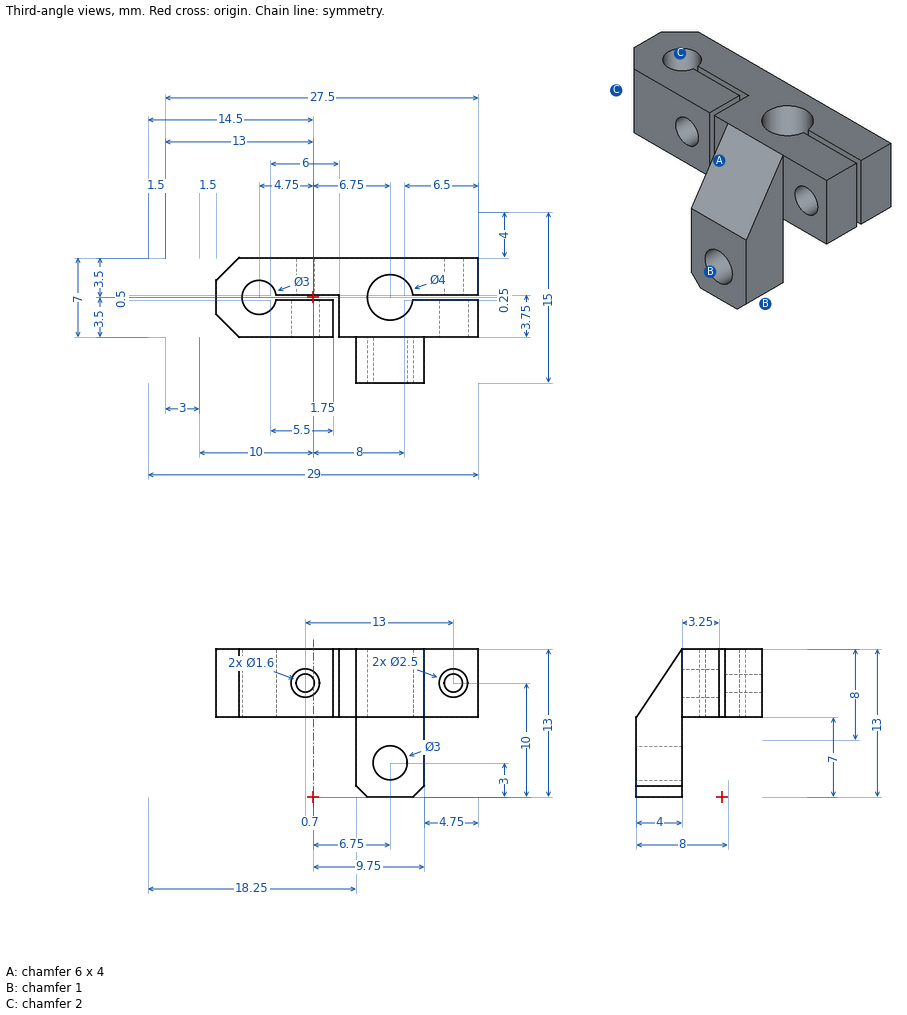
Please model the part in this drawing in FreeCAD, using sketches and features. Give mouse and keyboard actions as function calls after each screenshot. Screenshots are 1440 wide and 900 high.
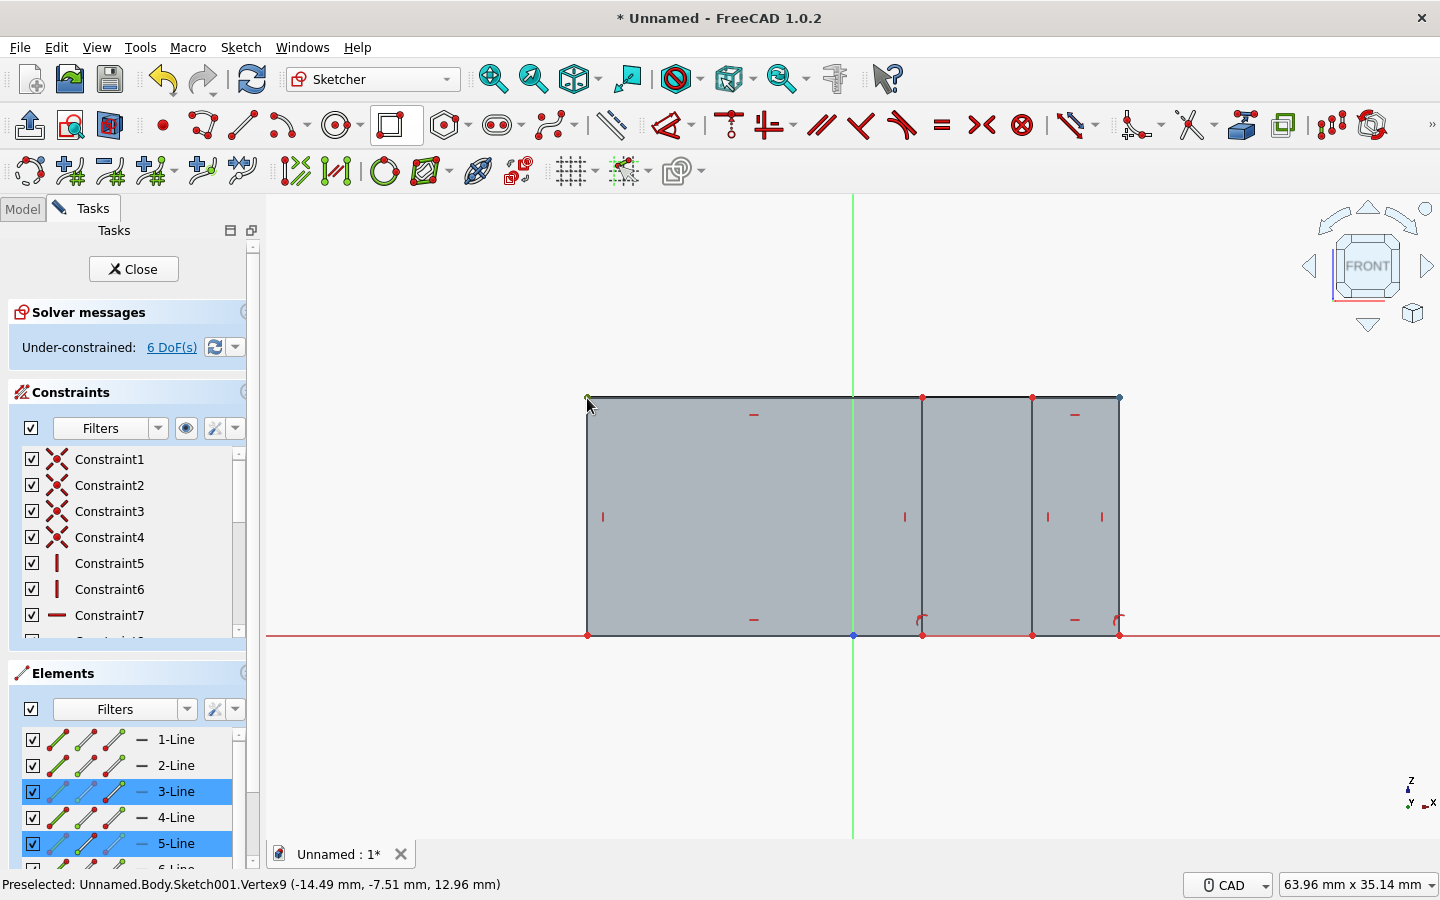
click(853, 769)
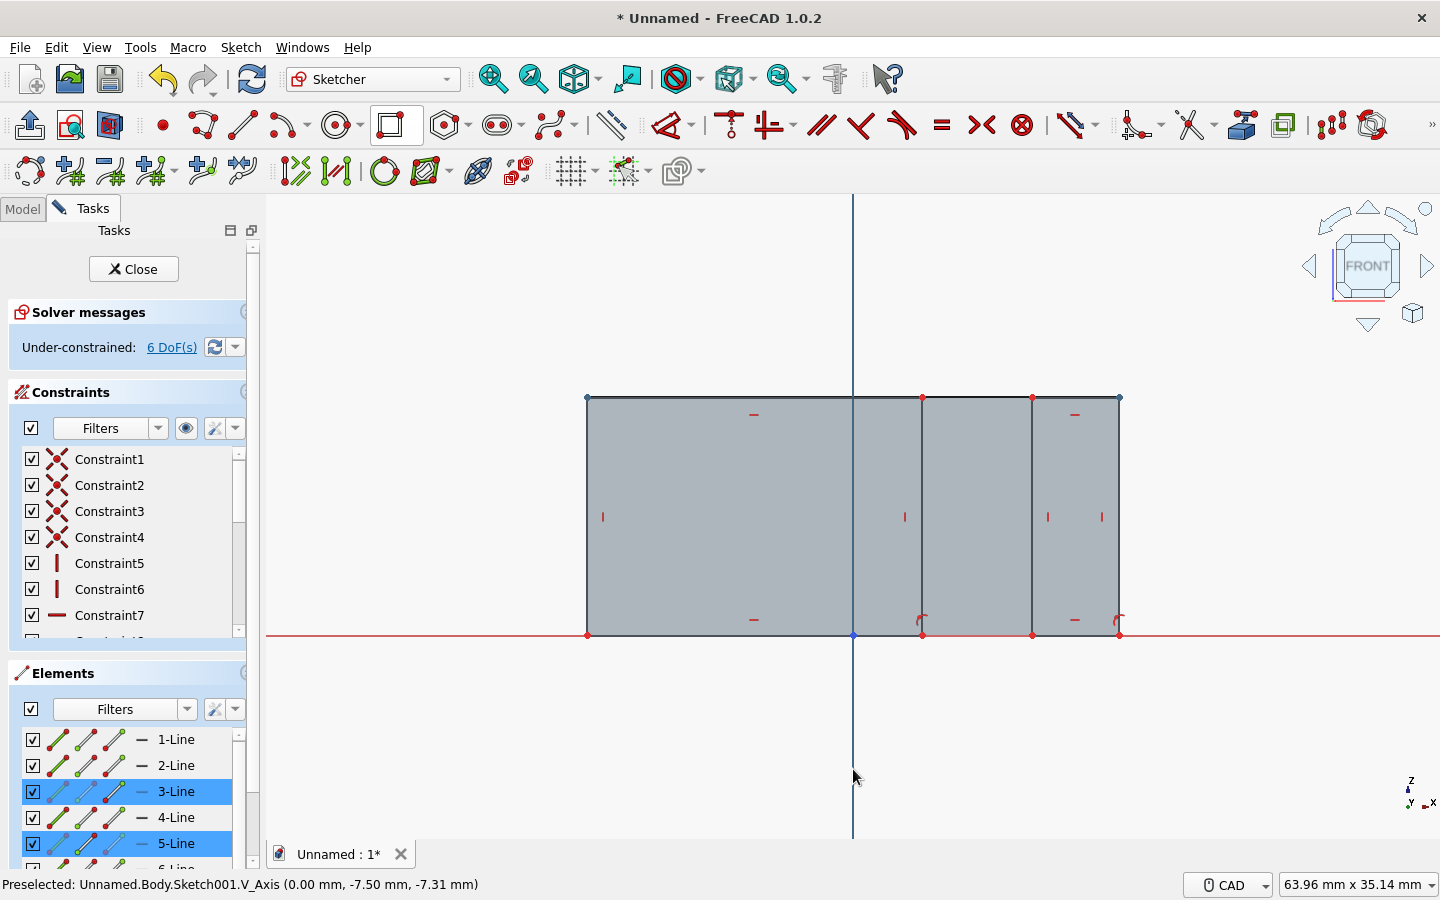
click(982, 126)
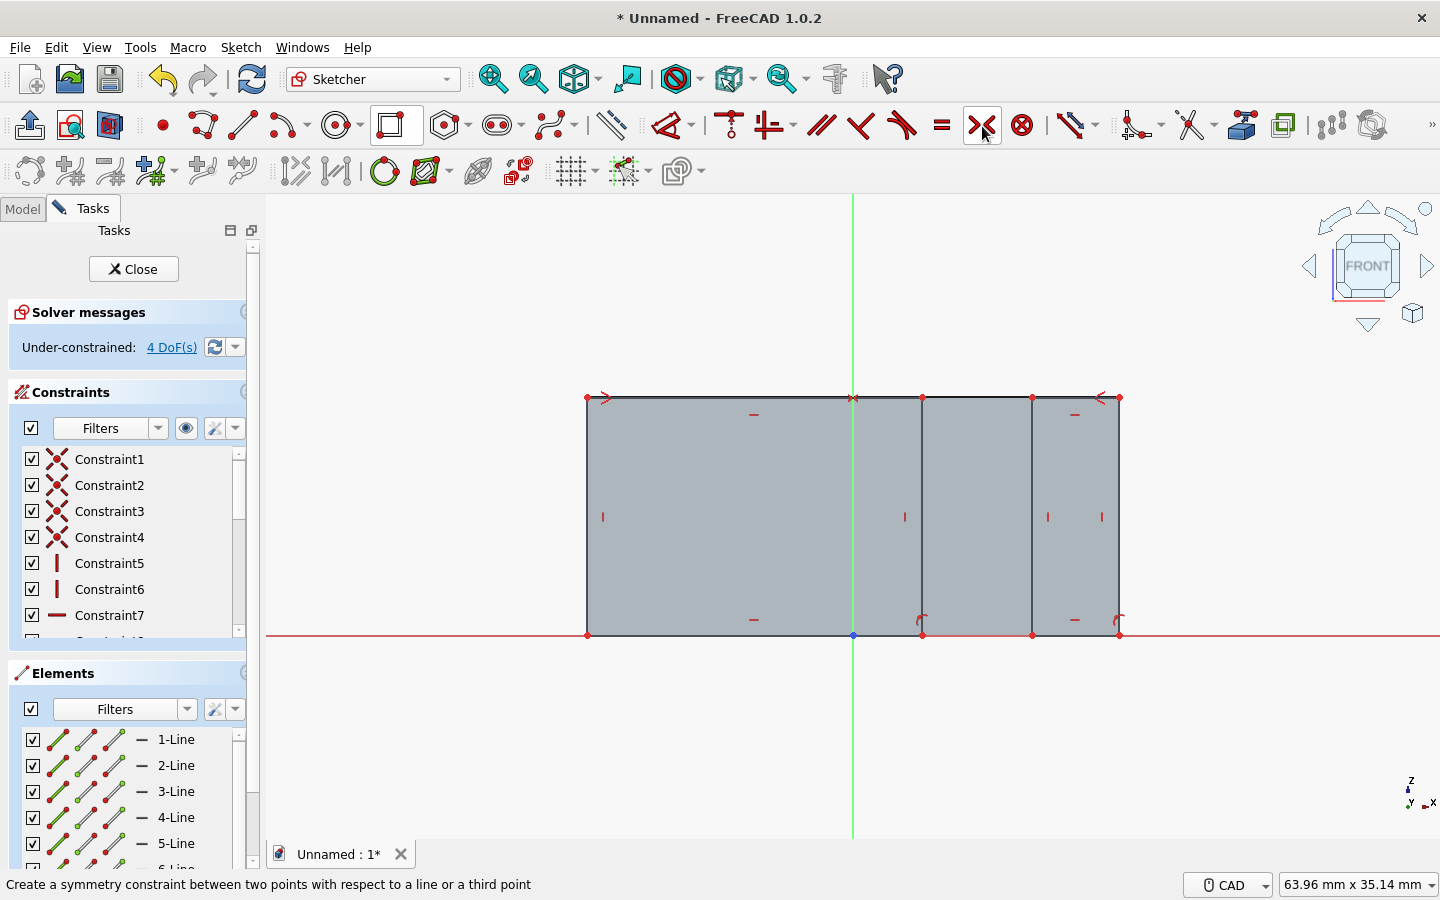
click(666, 126)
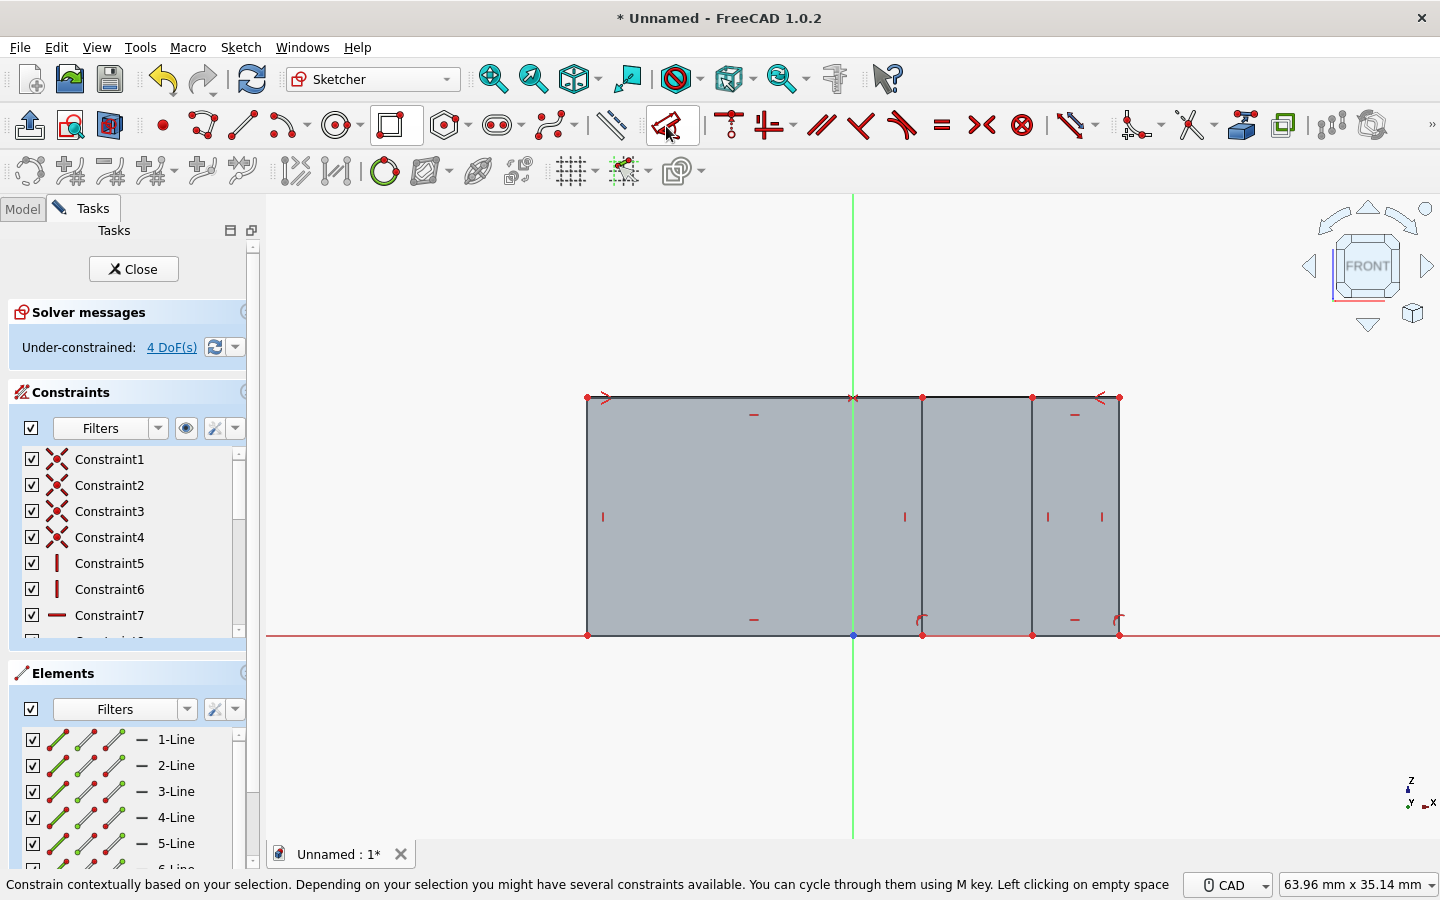
click(1032, 469)
click(1066, 517)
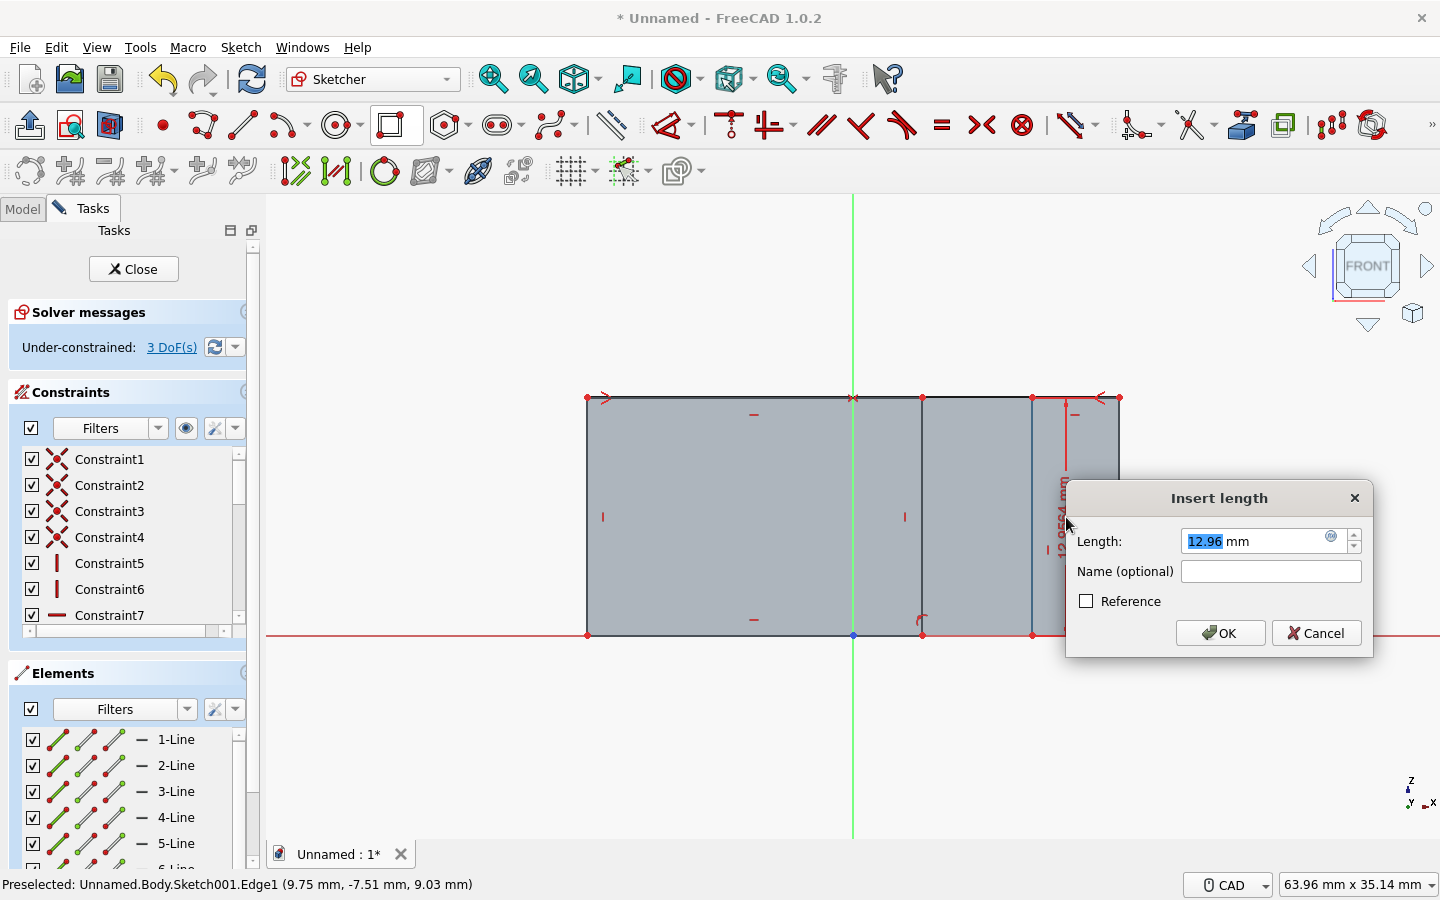
text(13)
key(Return)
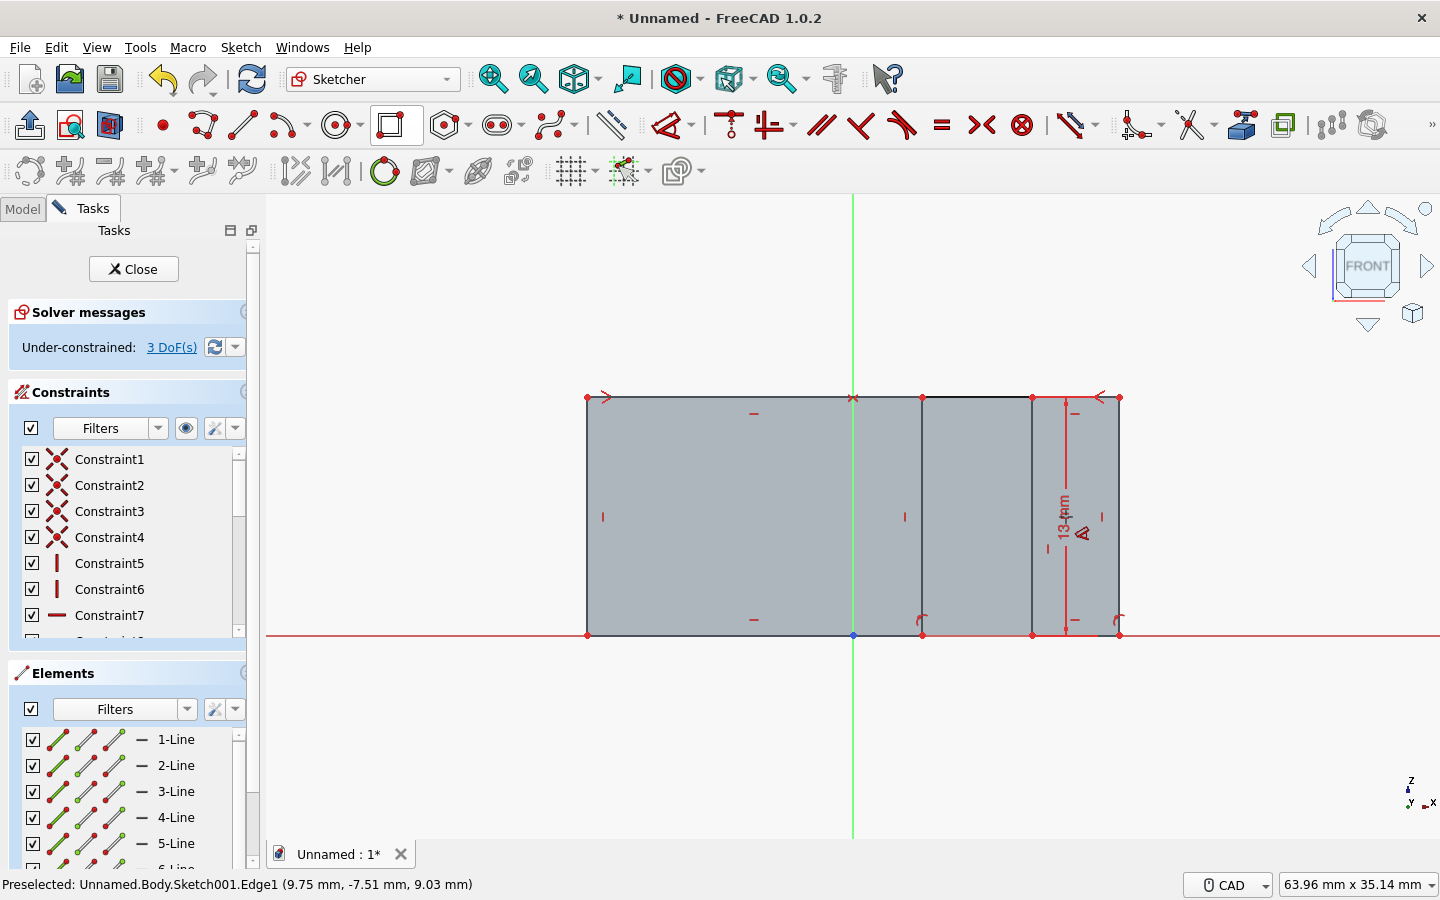
click(1058, 636)
click(1075, 670)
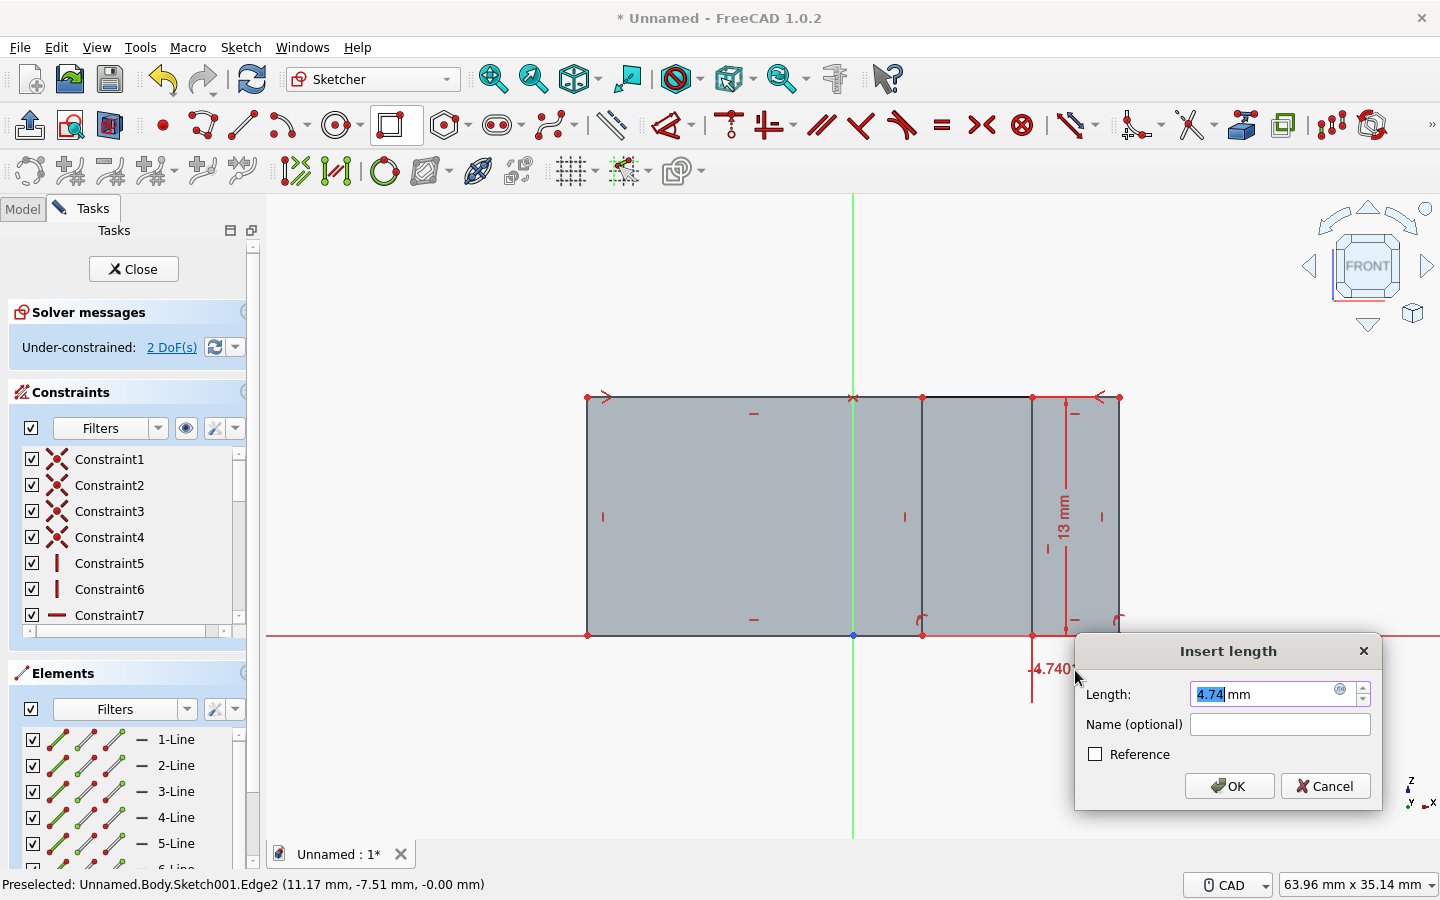
text(4.75)
key(Return)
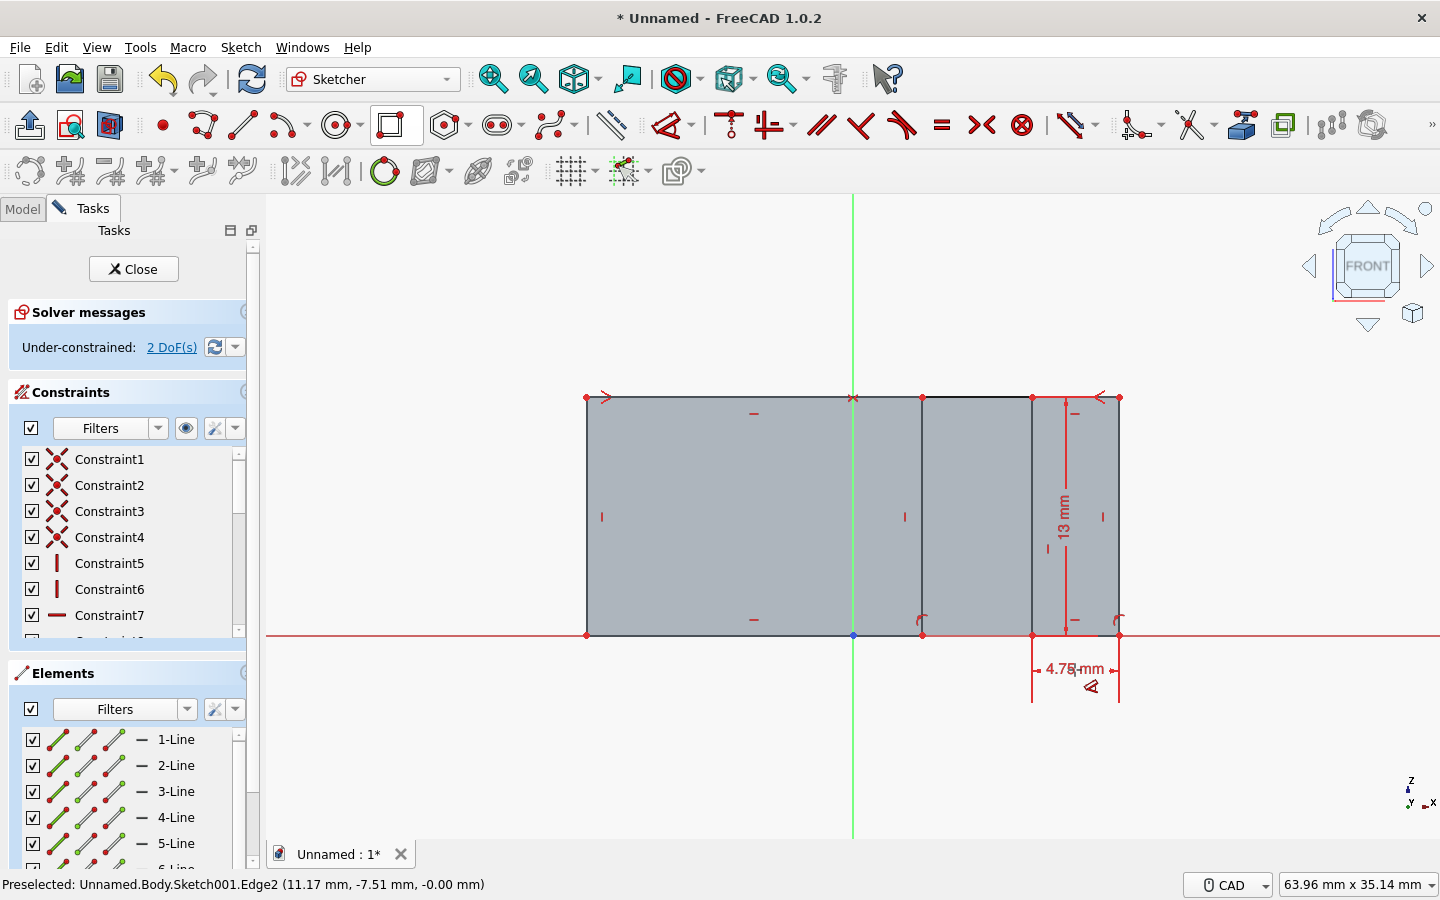
click(687, 636)
click(754, 670)